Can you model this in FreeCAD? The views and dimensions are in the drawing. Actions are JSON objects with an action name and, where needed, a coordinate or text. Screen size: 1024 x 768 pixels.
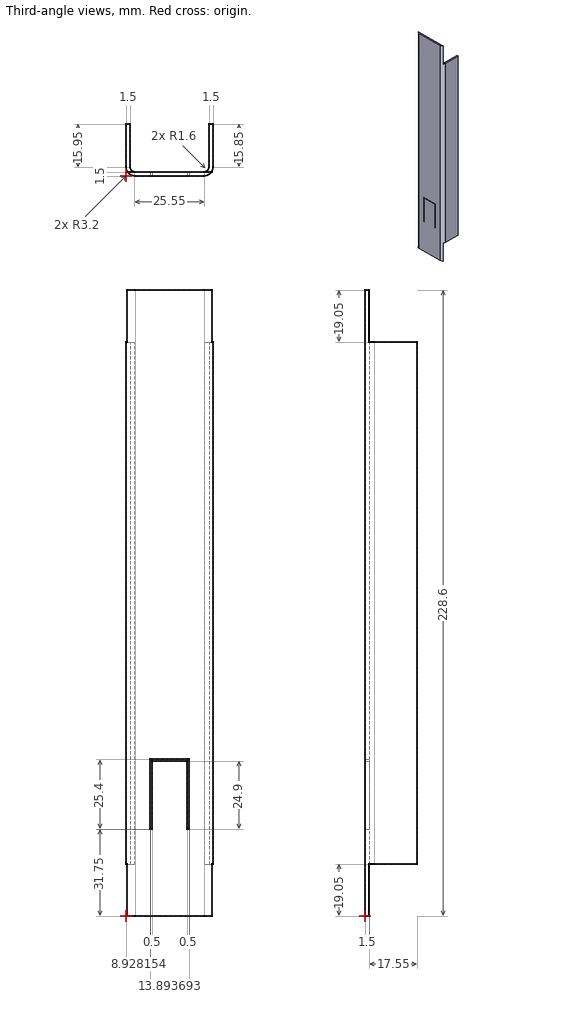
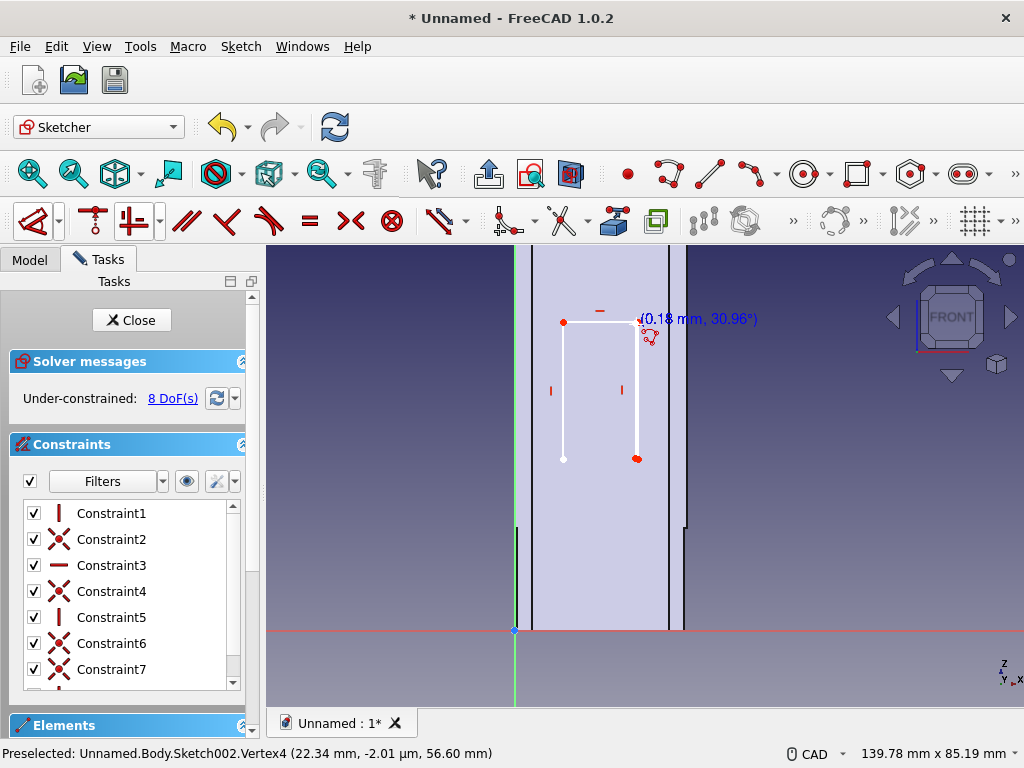
{"action": "scroll", "coordinate": [566, 324], "scroll_direction": "up", "scroll_amount": 9}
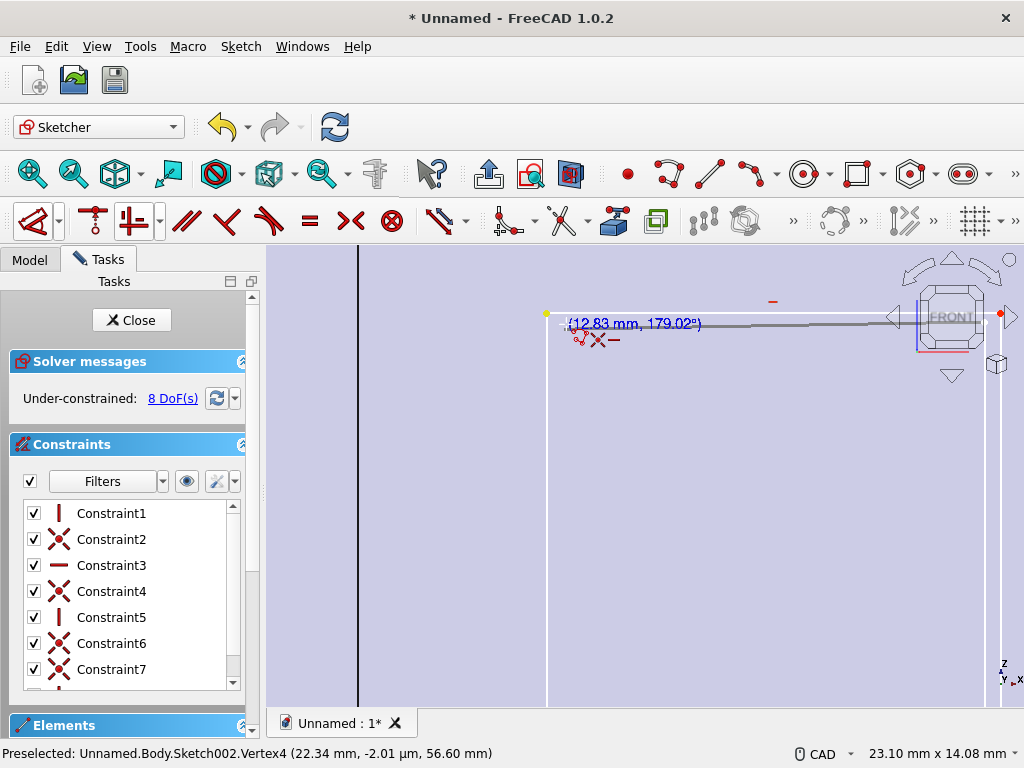
{"action": "left_click", "coordinate": [562, 321]}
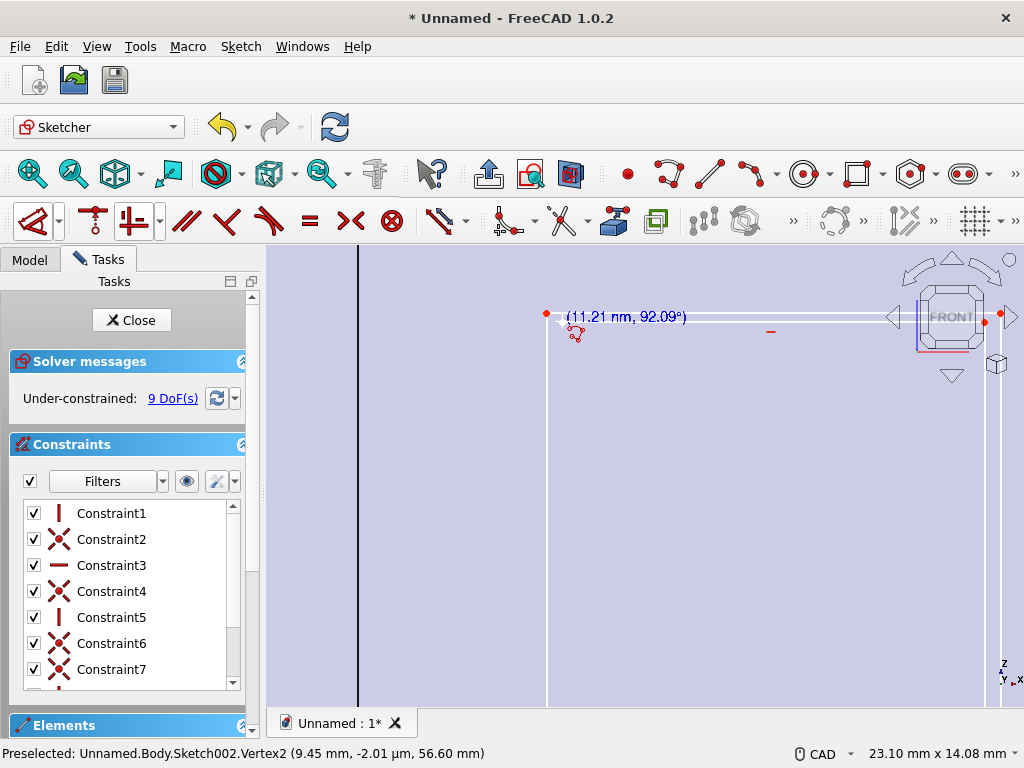
{"action": "scroll", "coordinate": [566, 324], "scroll_direction": "down", "scroll_amount": 9}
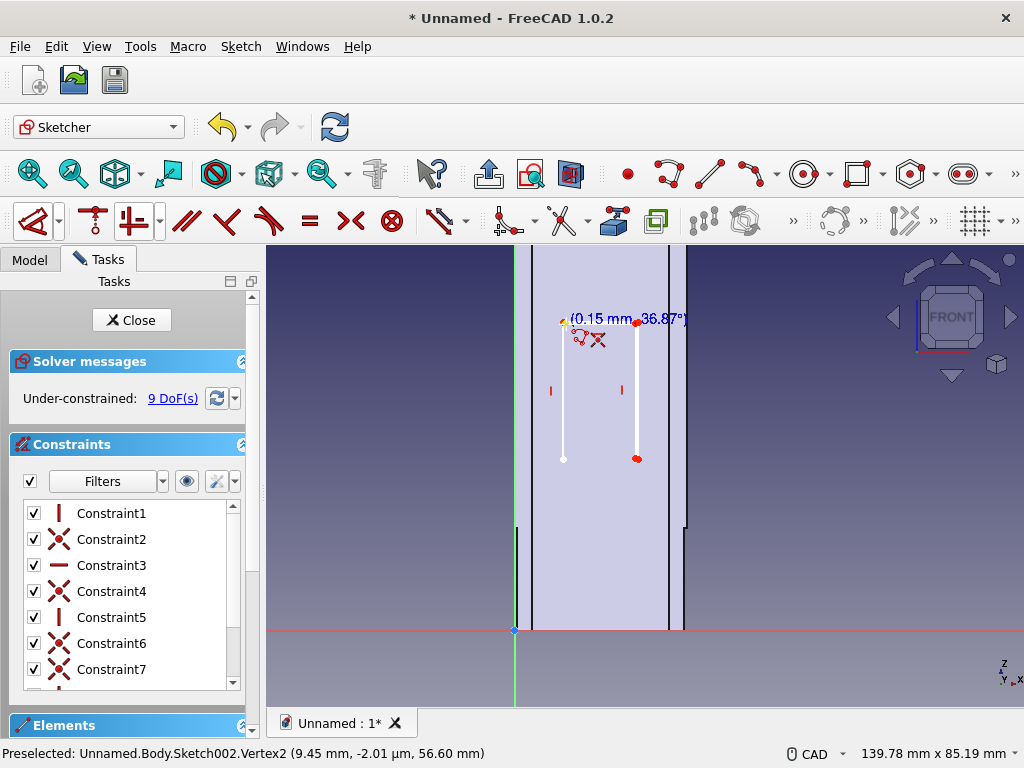
{"action": "scroll", "coordinate": [566, 459], "scroll_direction": "up", "scroll_amount": 9}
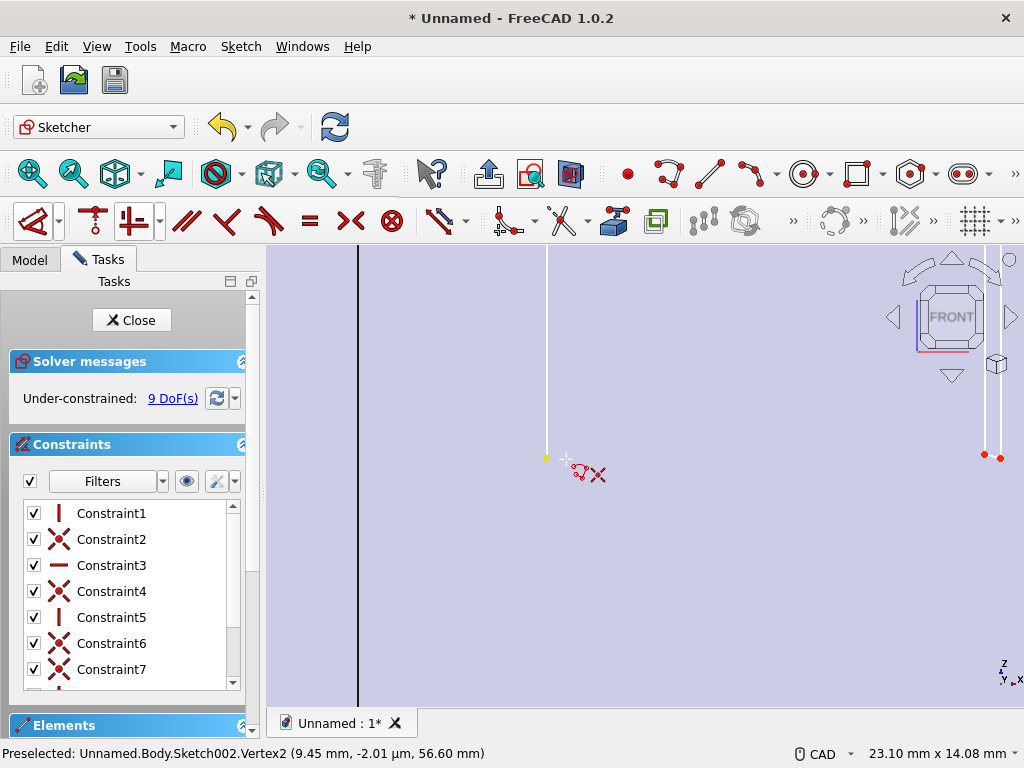
{"action": "left_click", "coordinate": [562, 455]}
{"action": "left_click", "coordinate": [547, 459]}
{"action": "key", "text": "Escape"}
{"action": "key", "text": "Escape"}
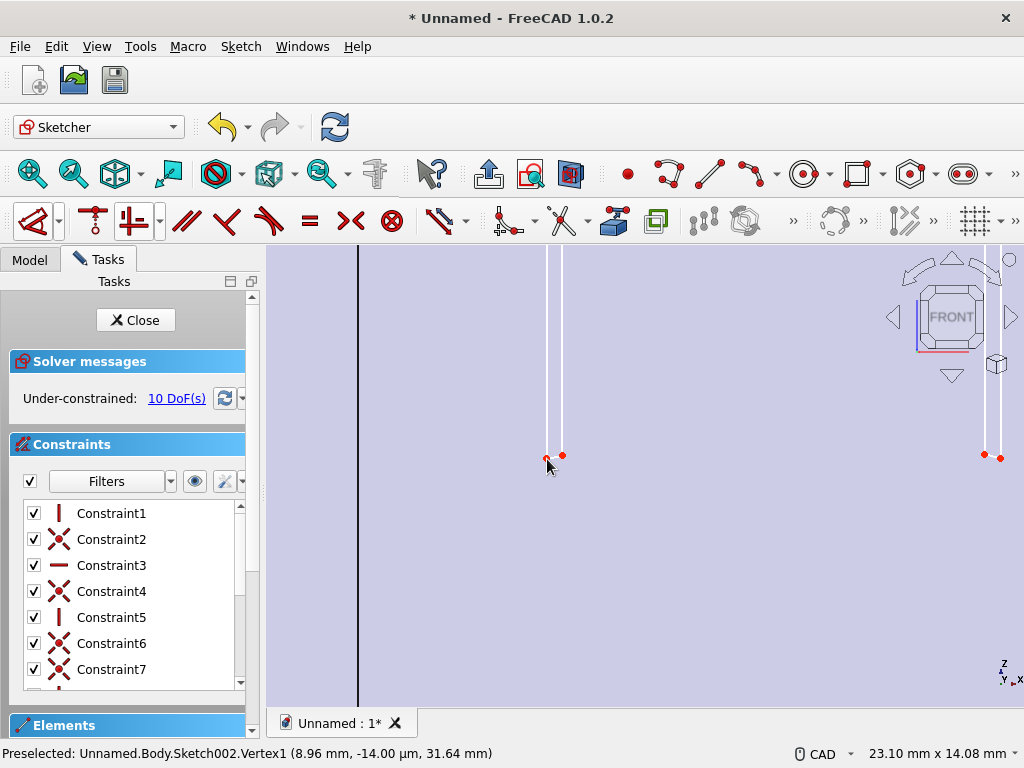
{"action": "scroll", "coordinate": [566, 460], "scroll_direction": "down", "scroll_amount": 9}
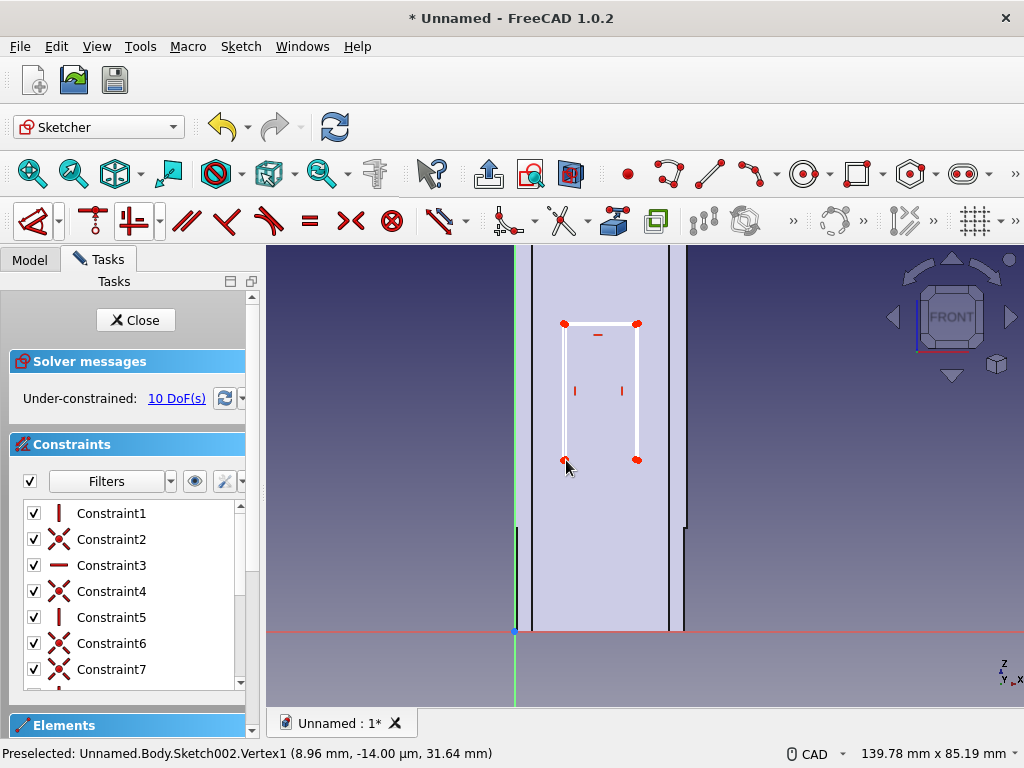
{"action": "scroll", "coordinate": [637, 460], "scroll_direction": "up", "scroll_amount": 12}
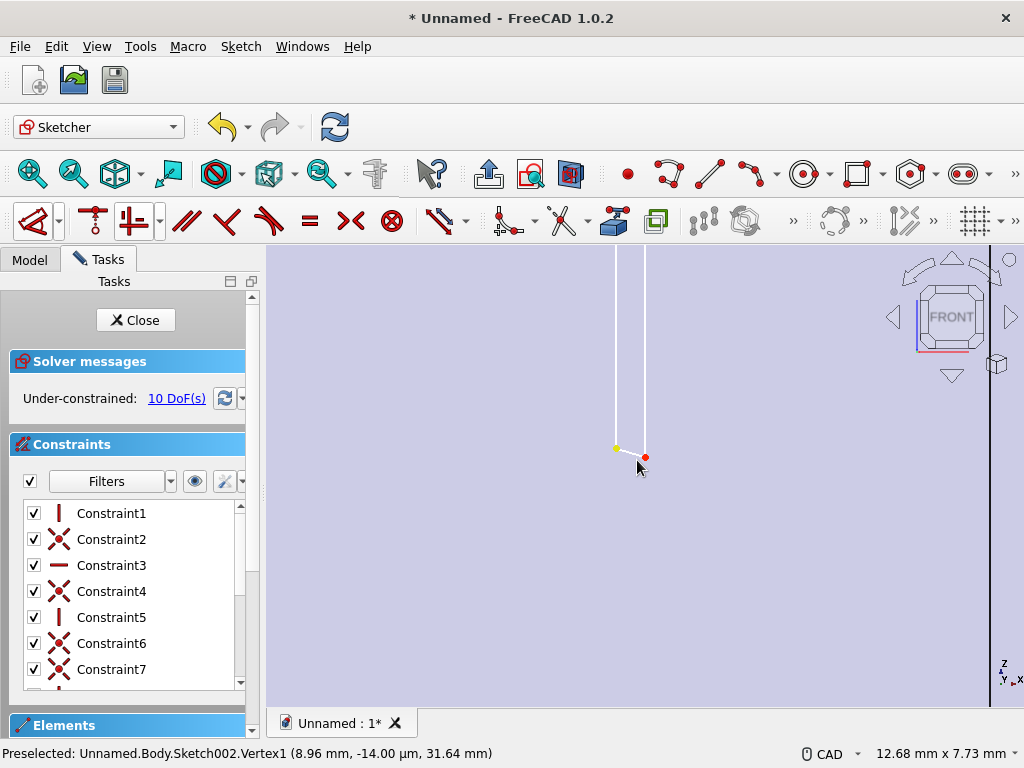
{"action": "left_click", "coordinate": [631, 453]}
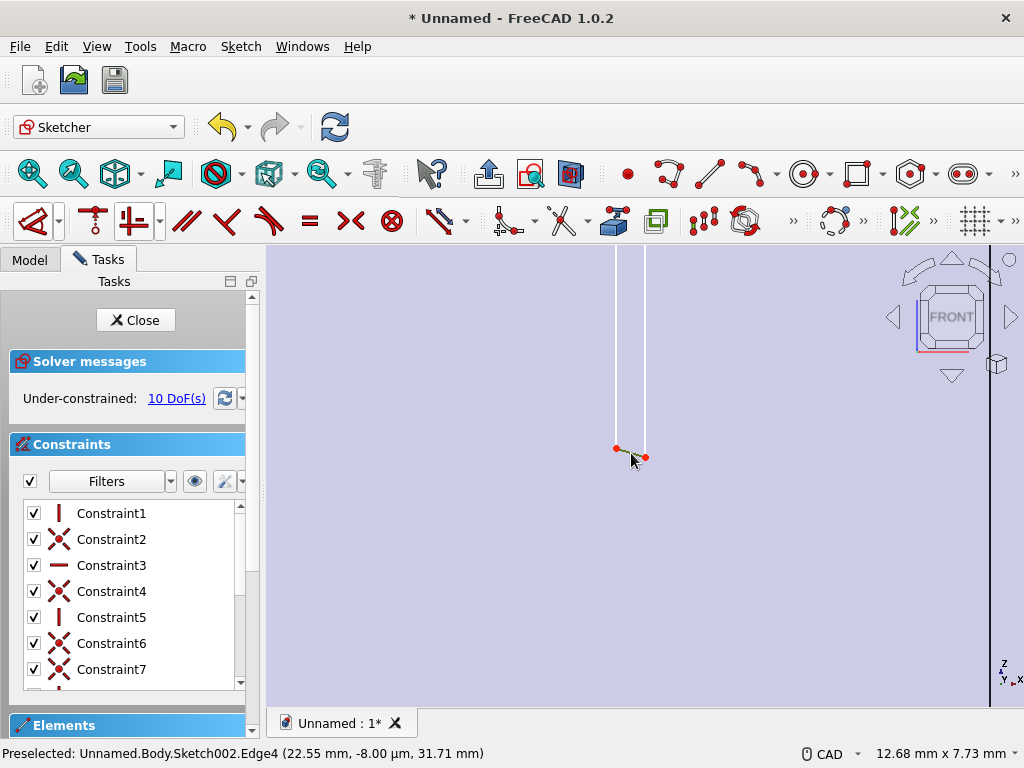
{"action": "left_click", "coordinate": [160, 222]}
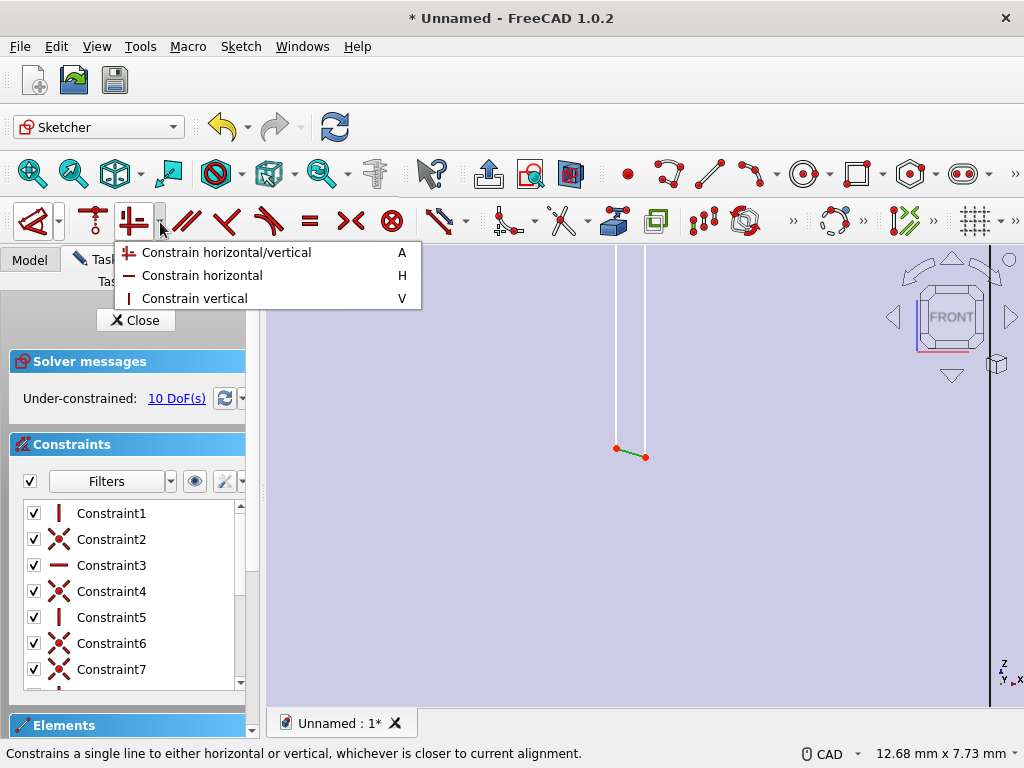
{"action": "left_click", "coordinate": [268, 276]}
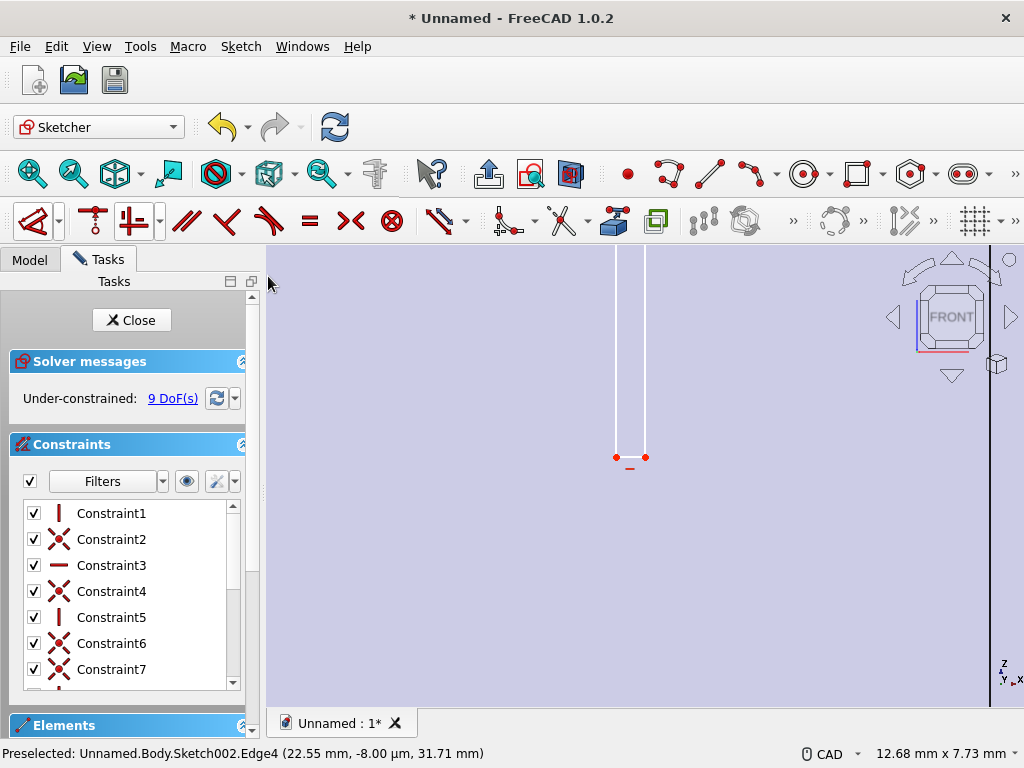
{"action": "scroll", "coordinate": [637, 460], "scroll_direction": "down", "scroll_amount": 12}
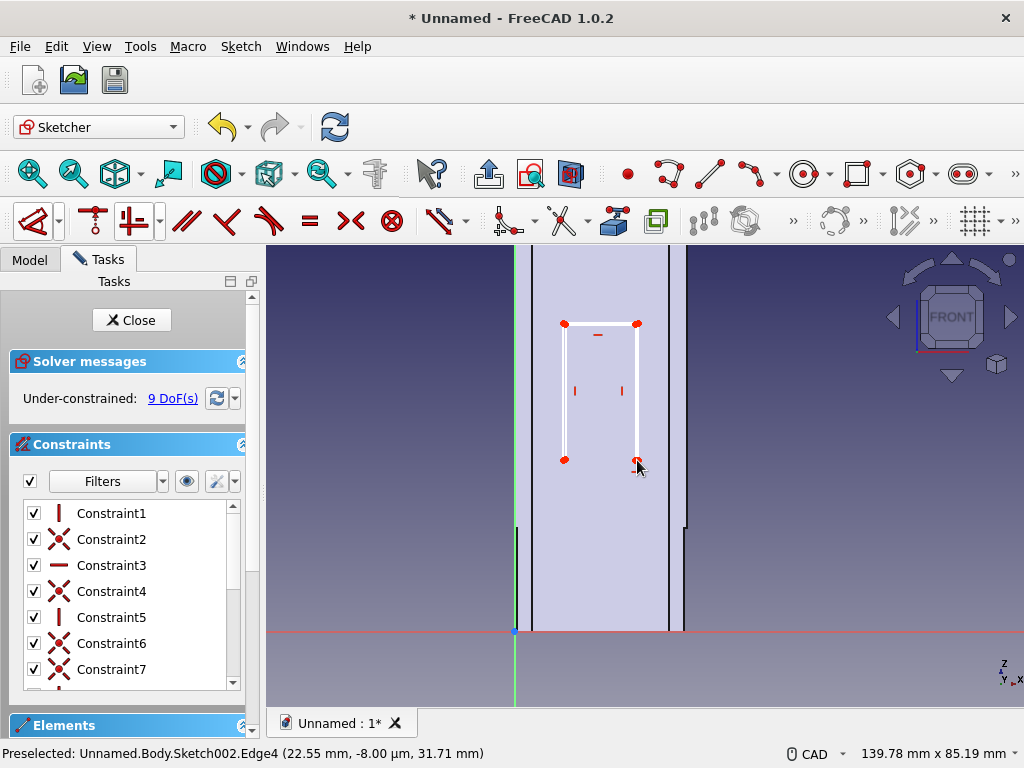
{"action": "scroll", "coordinate": [565, 460], "scroll_direction": "up", "scroll_amount": 14}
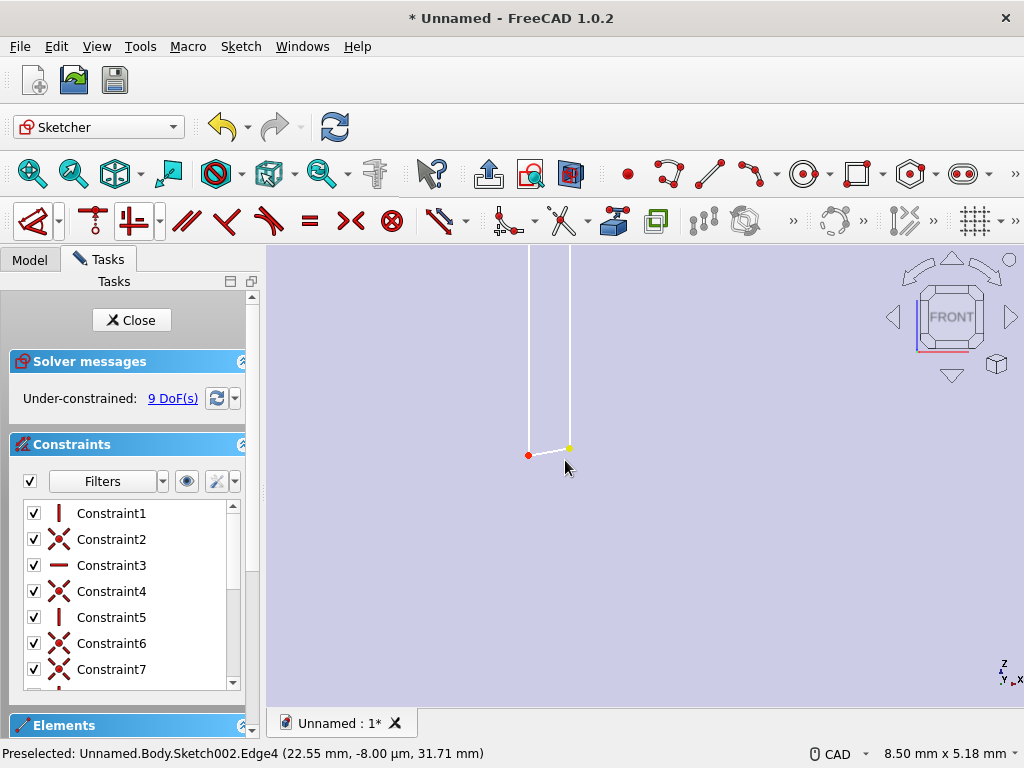
{"action": "left_click", "coordinate": [554, 451]}